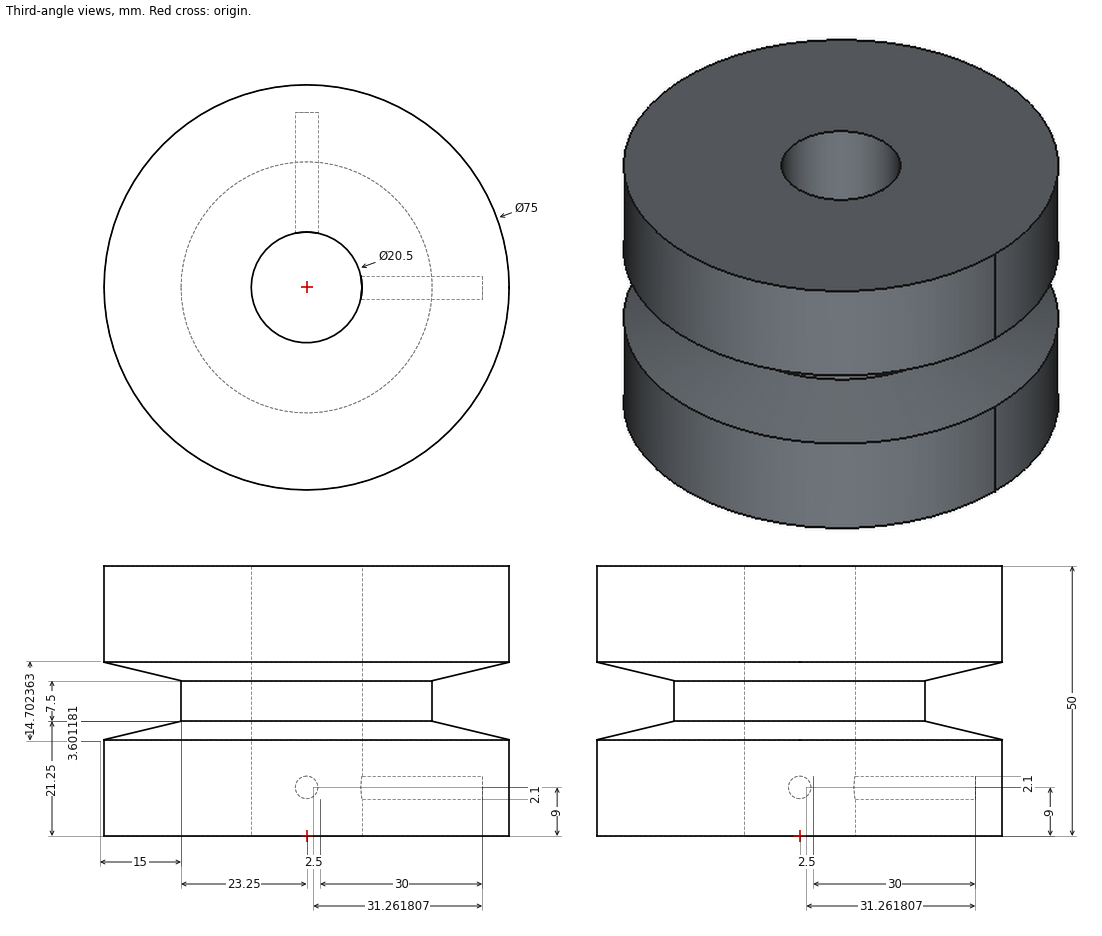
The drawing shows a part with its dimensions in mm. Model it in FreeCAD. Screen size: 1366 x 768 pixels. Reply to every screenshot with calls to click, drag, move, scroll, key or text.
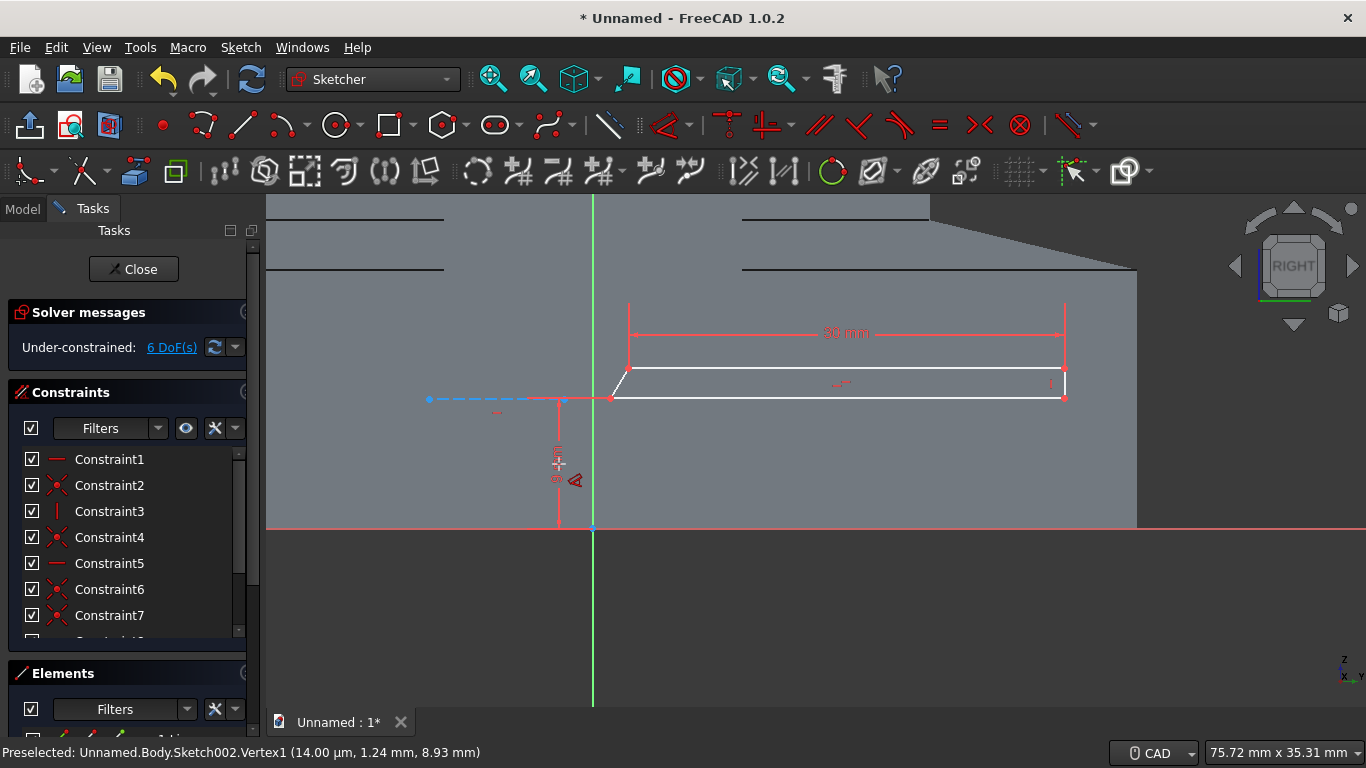
click(565, 399)
click(531, 434)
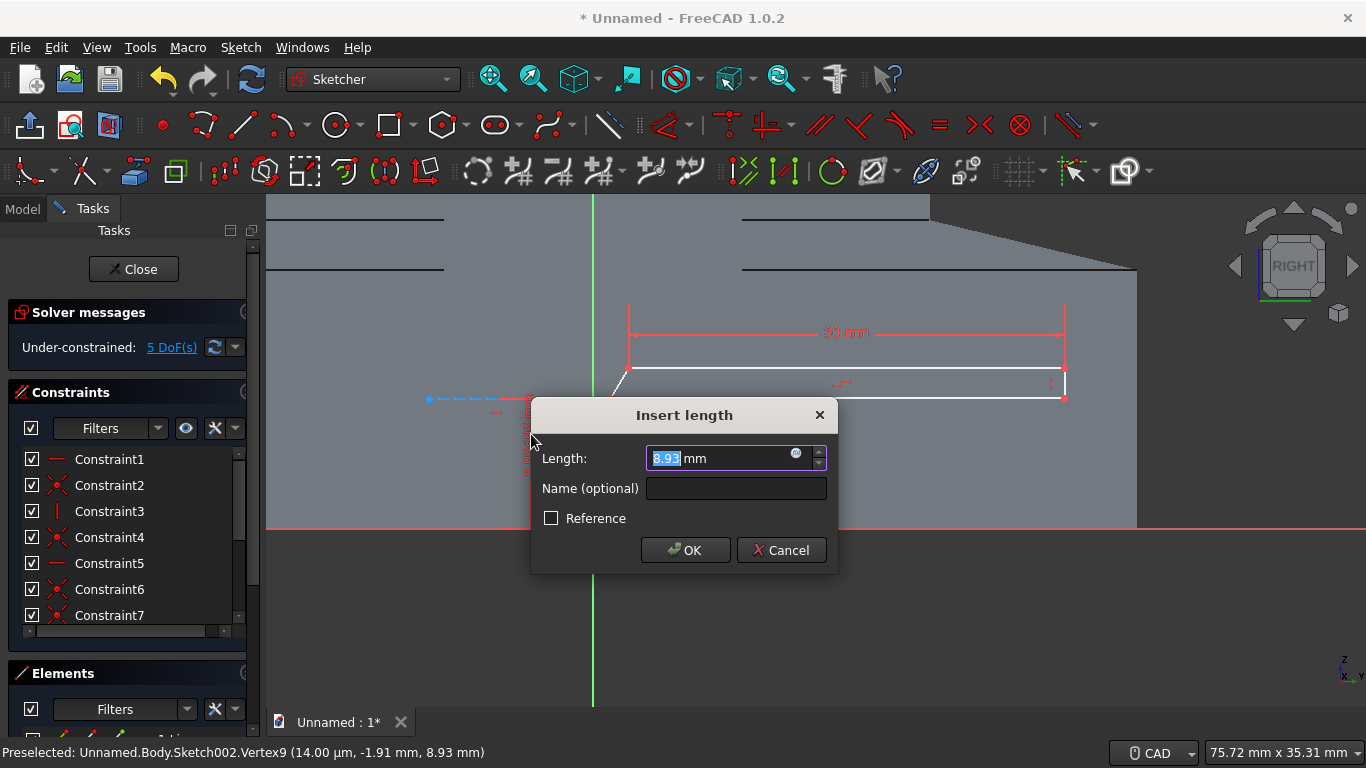
text(9)
key(Return)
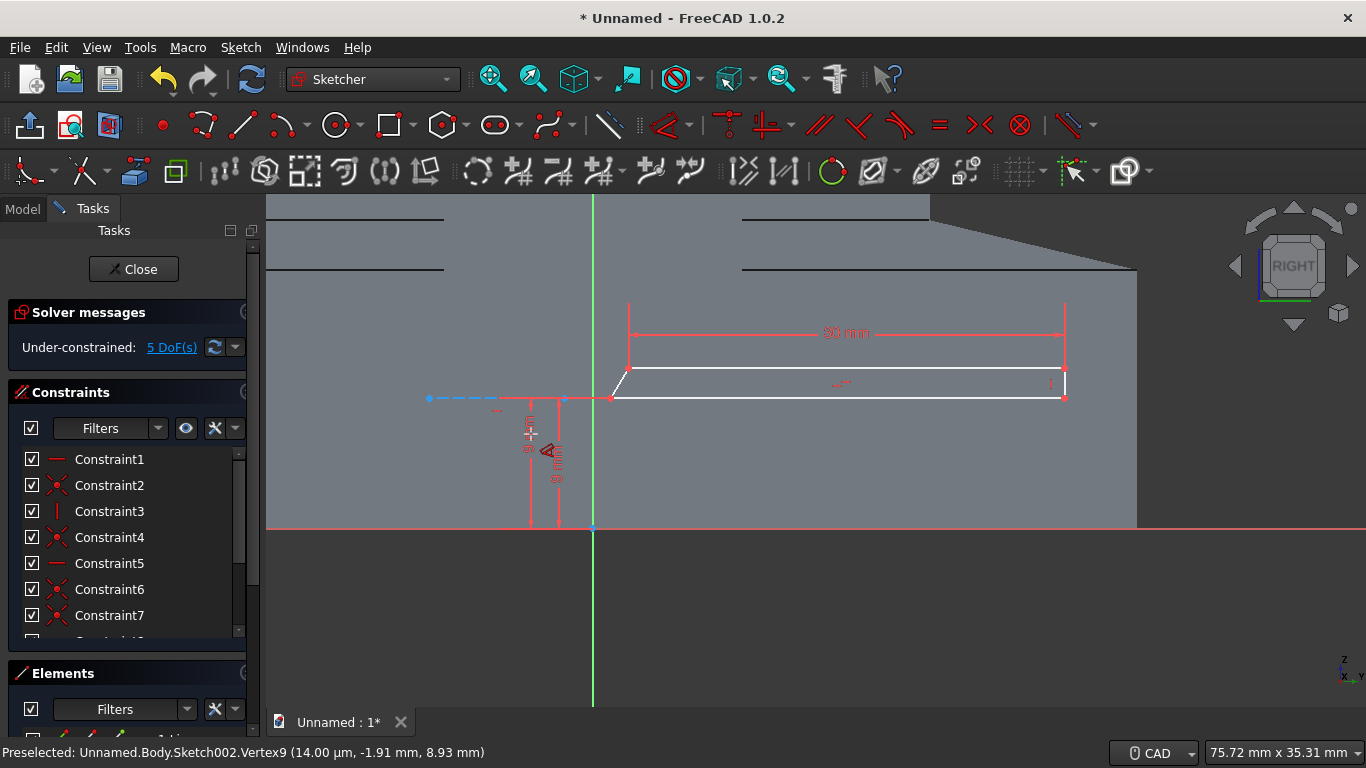
scroll(1065, 386, up, 2)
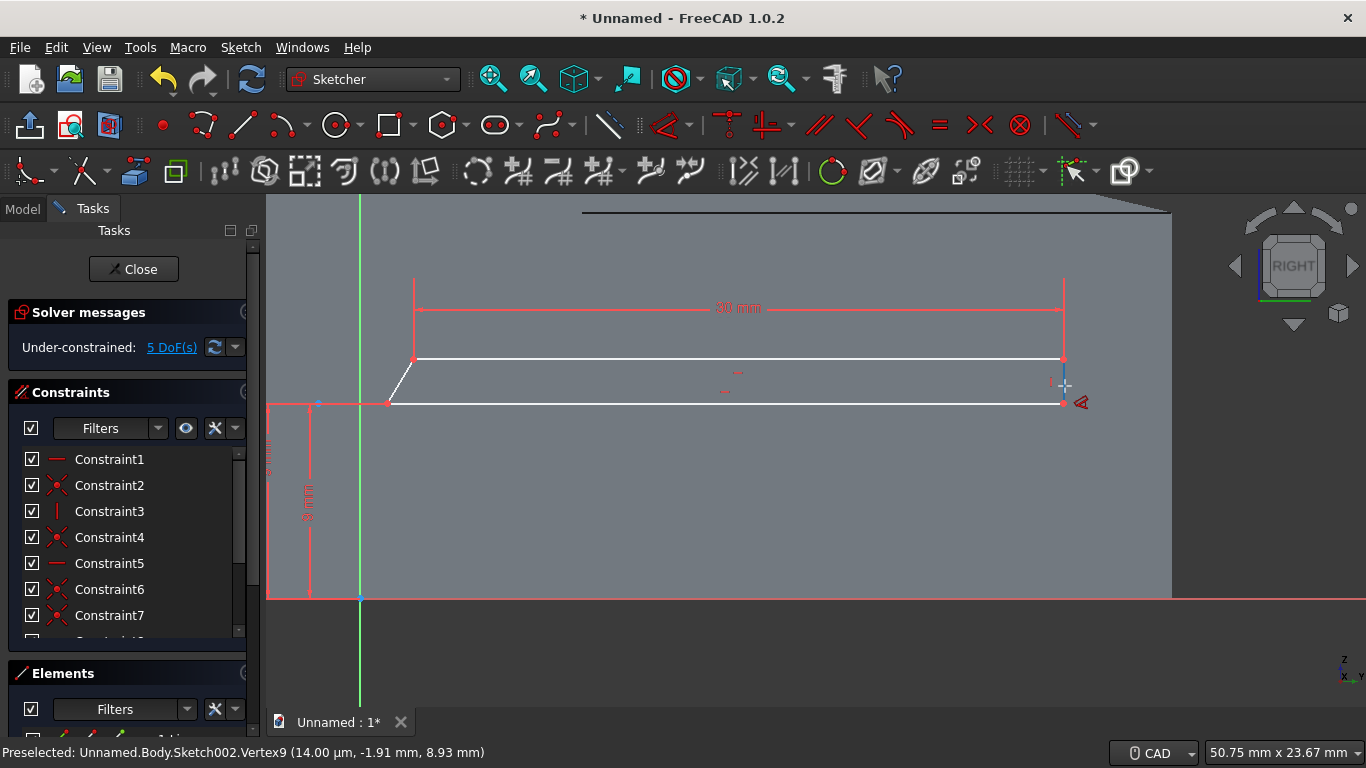
click(1064, 386)
click(1098, 382)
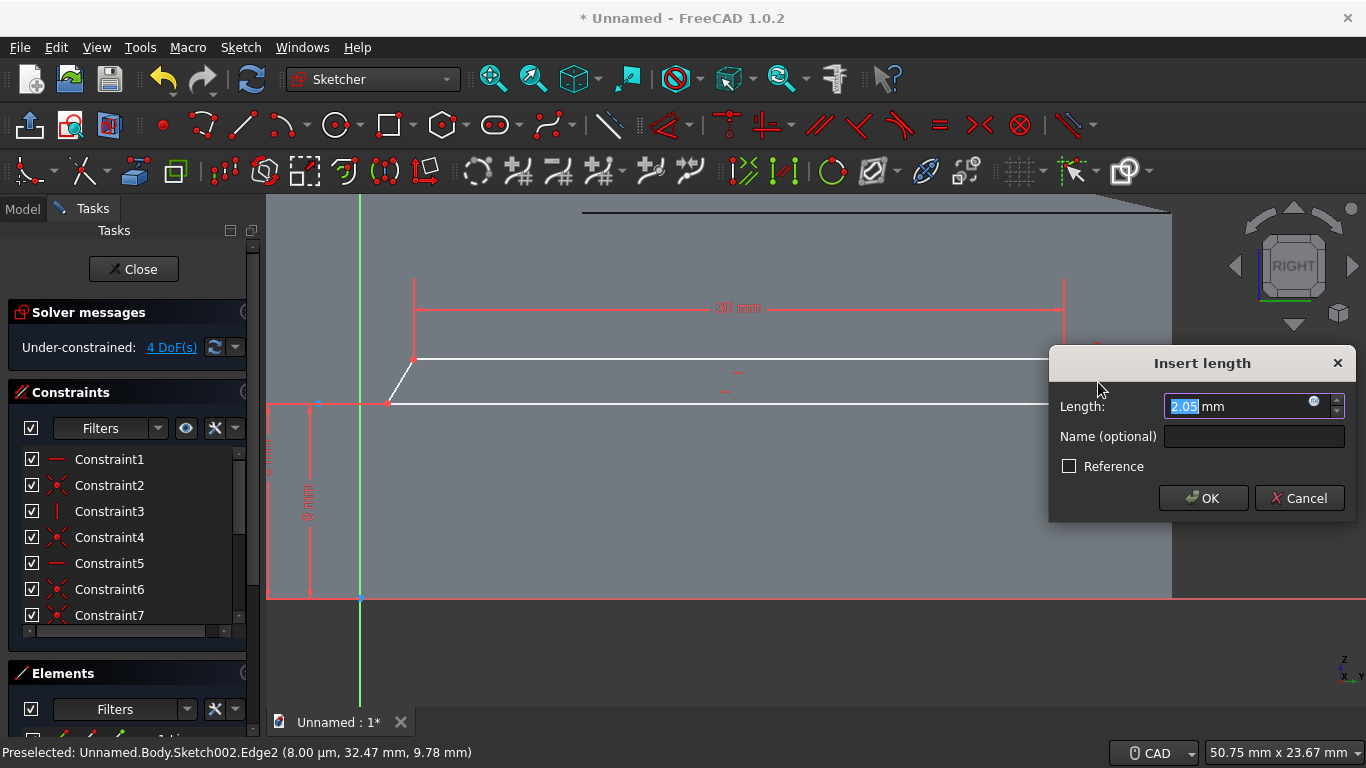
text(2.1)
key(Return)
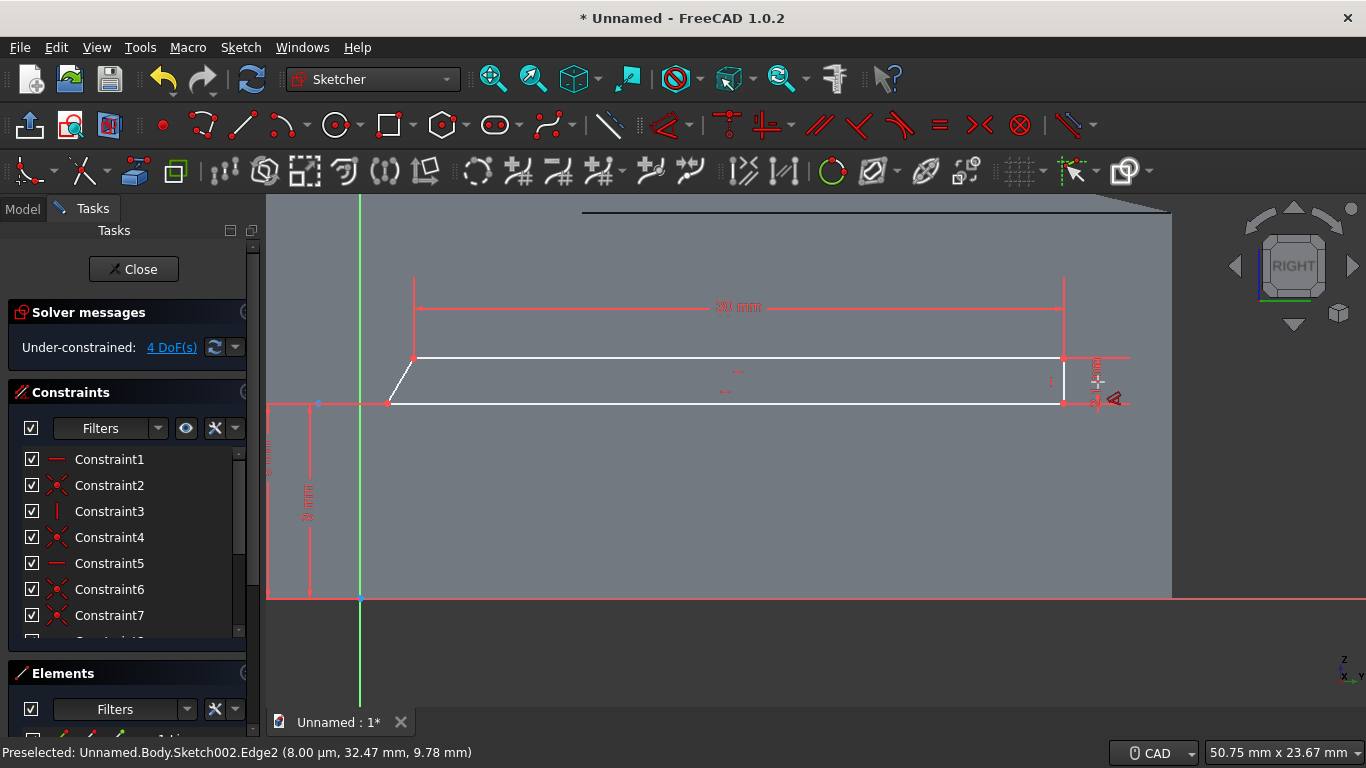
click(414, 358)
click(387, 633)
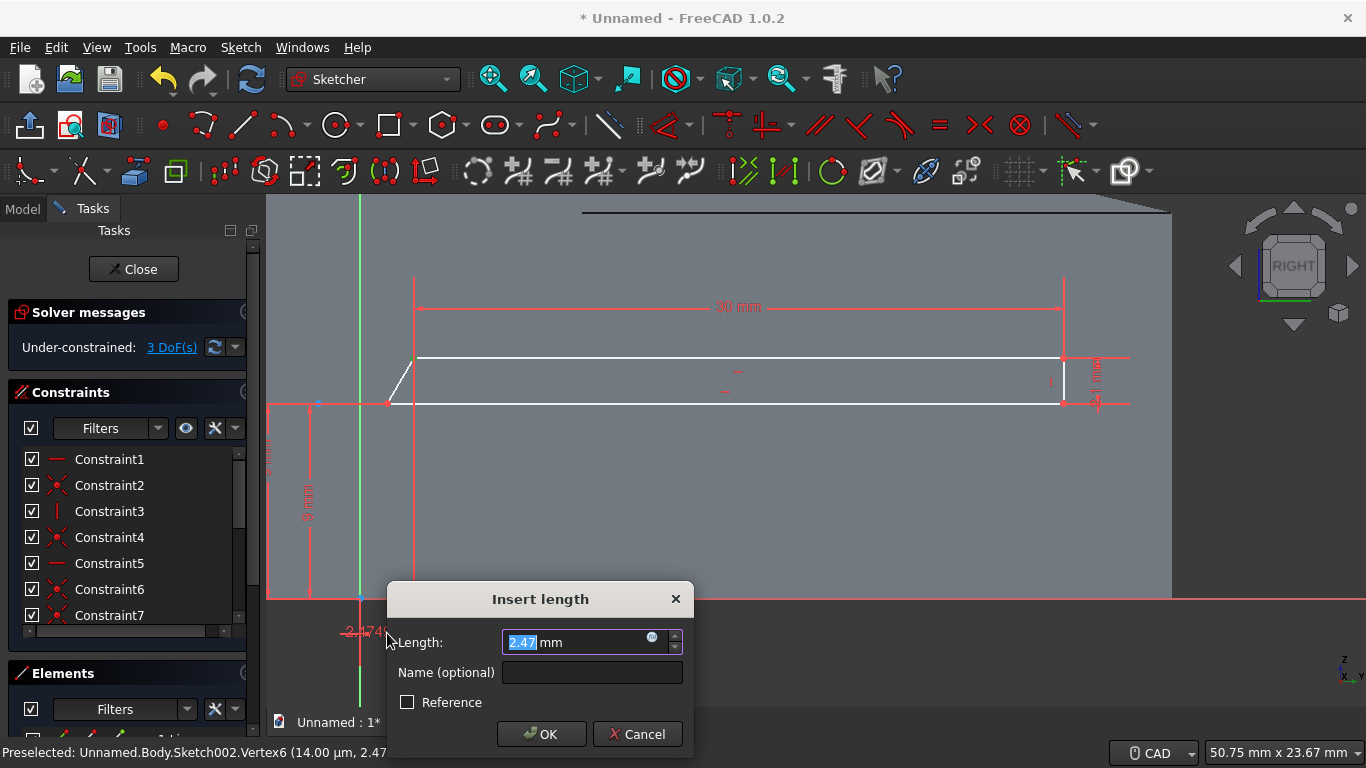
text(2.5)
key(Return)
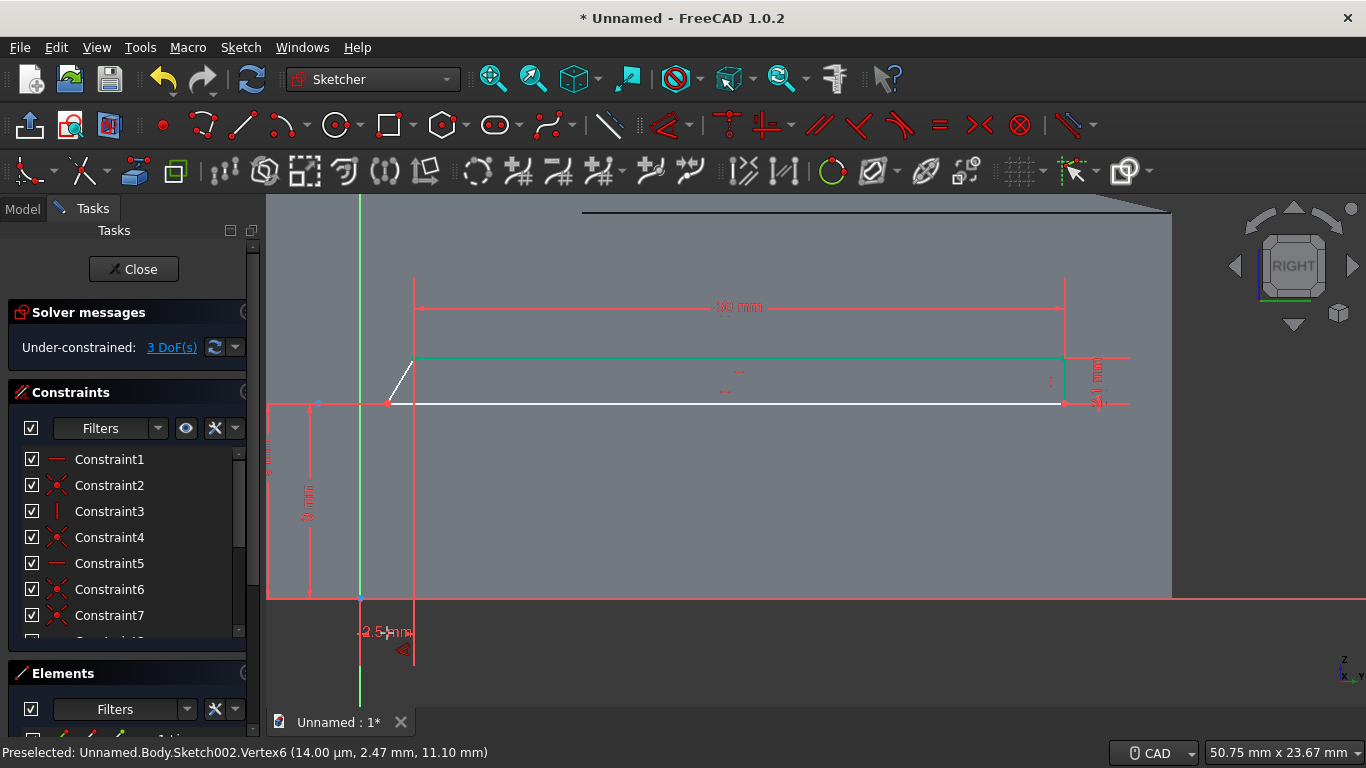
click(590, 404)
click(726, 438)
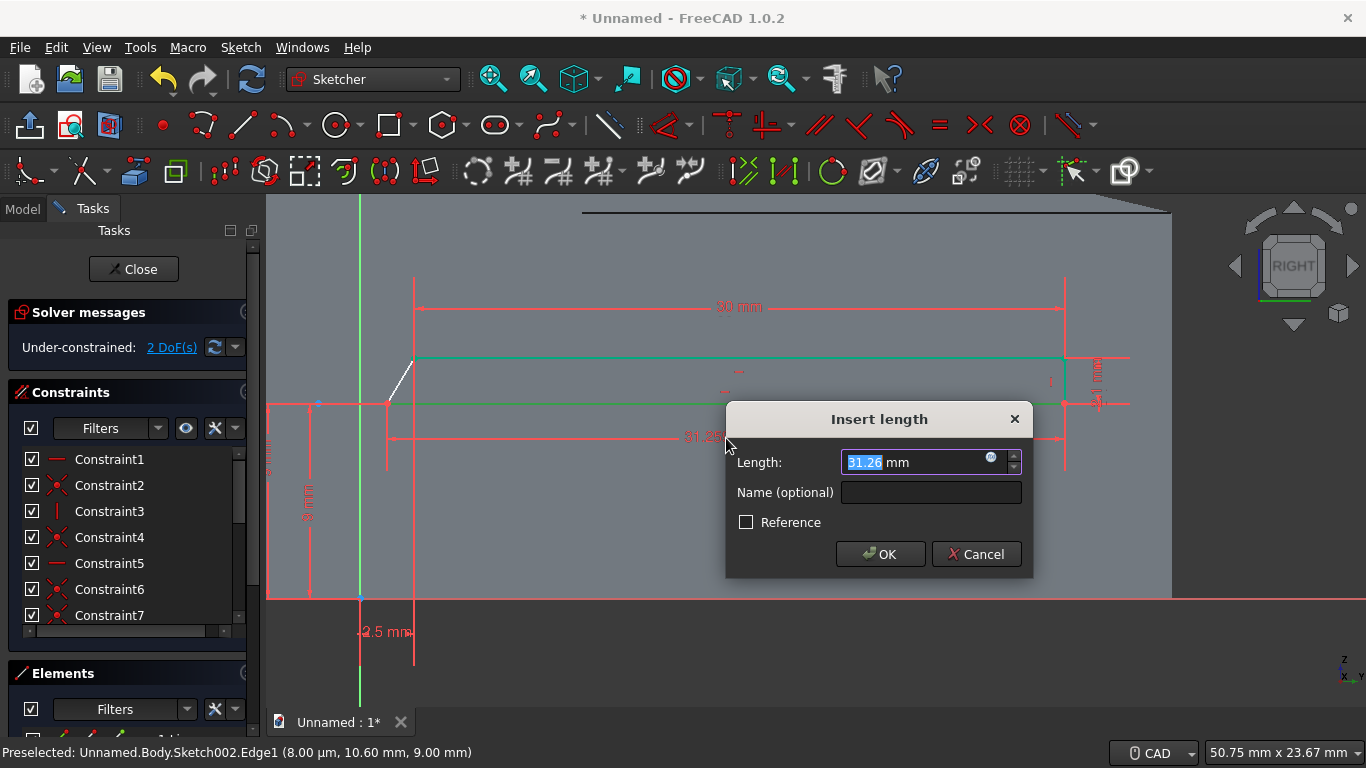
text(31.261807)
key(Return)
key(Escape)